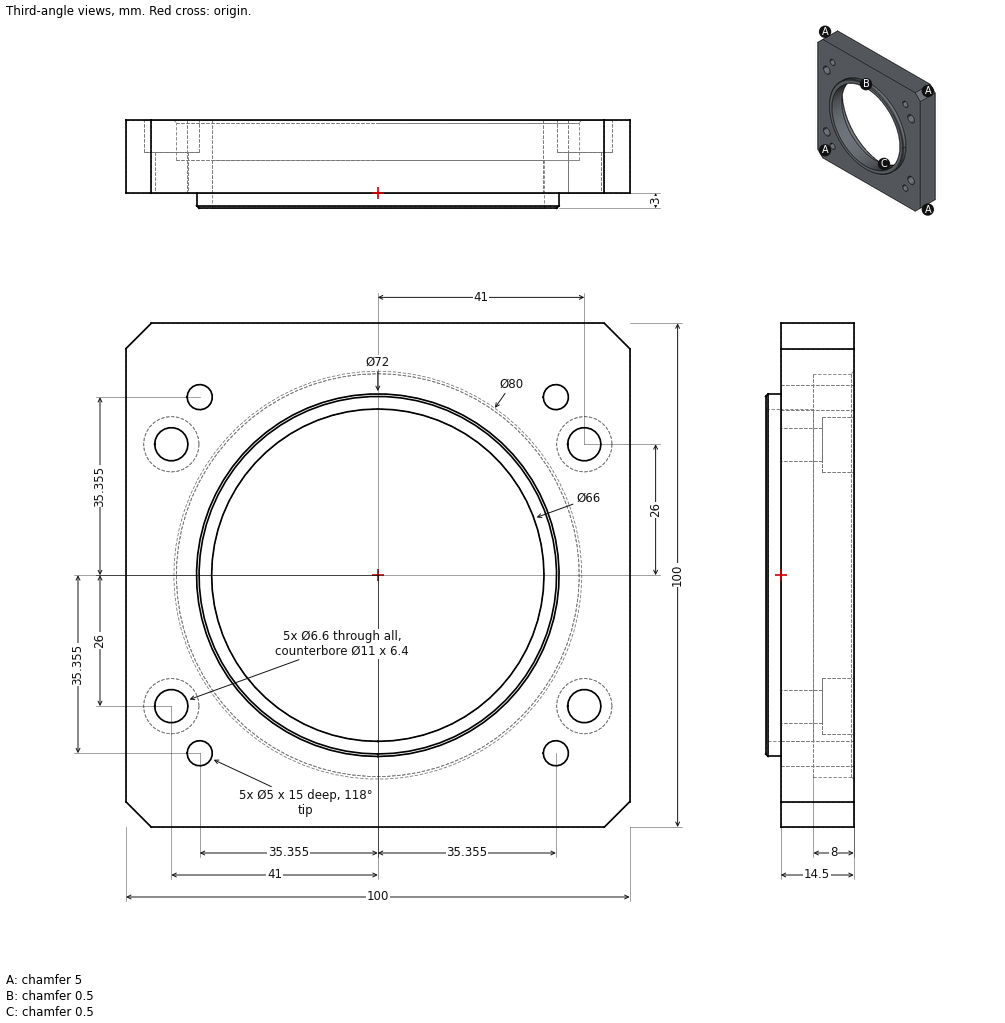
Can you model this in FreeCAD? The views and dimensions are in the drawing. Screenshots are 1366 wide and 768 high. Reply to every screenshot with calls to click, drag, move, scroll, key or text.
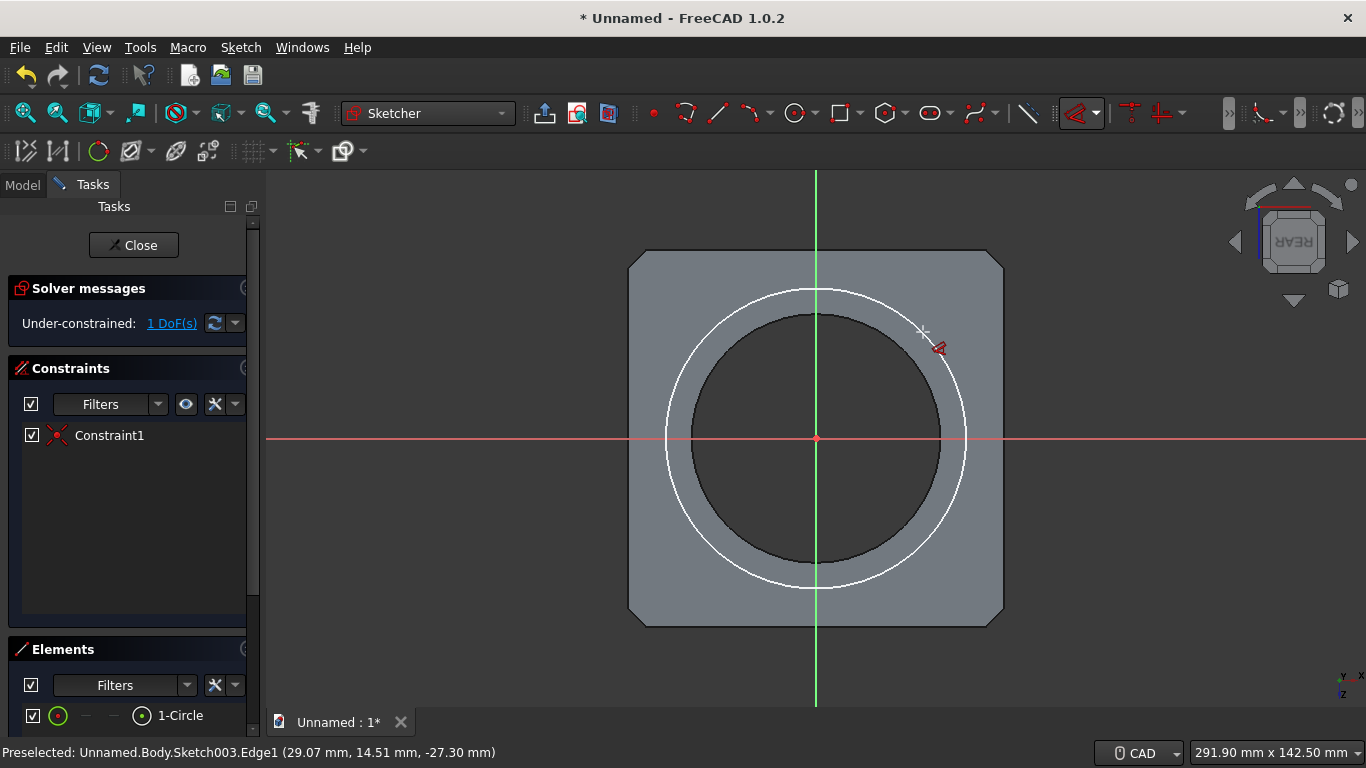
click(922, 332)
click(945, 309)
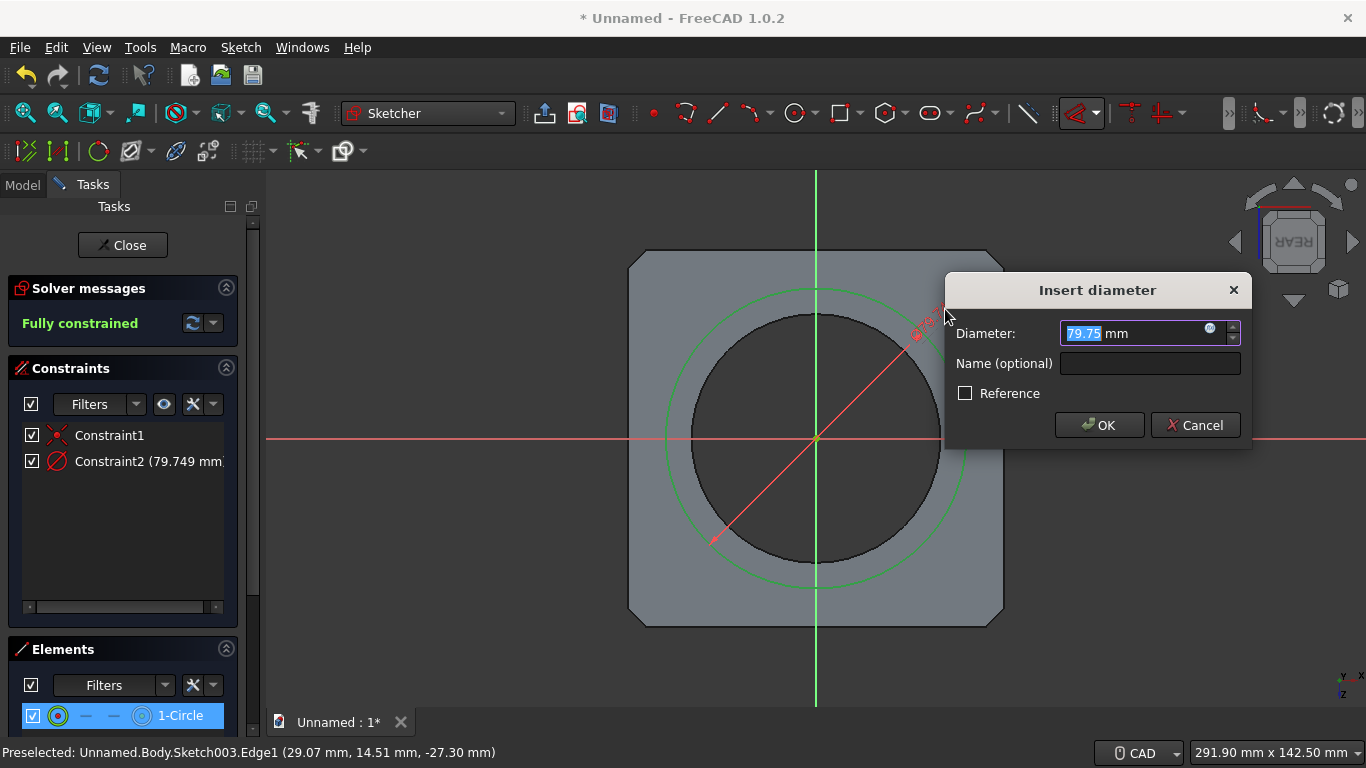
text(80)
key(Return)
key(Escape)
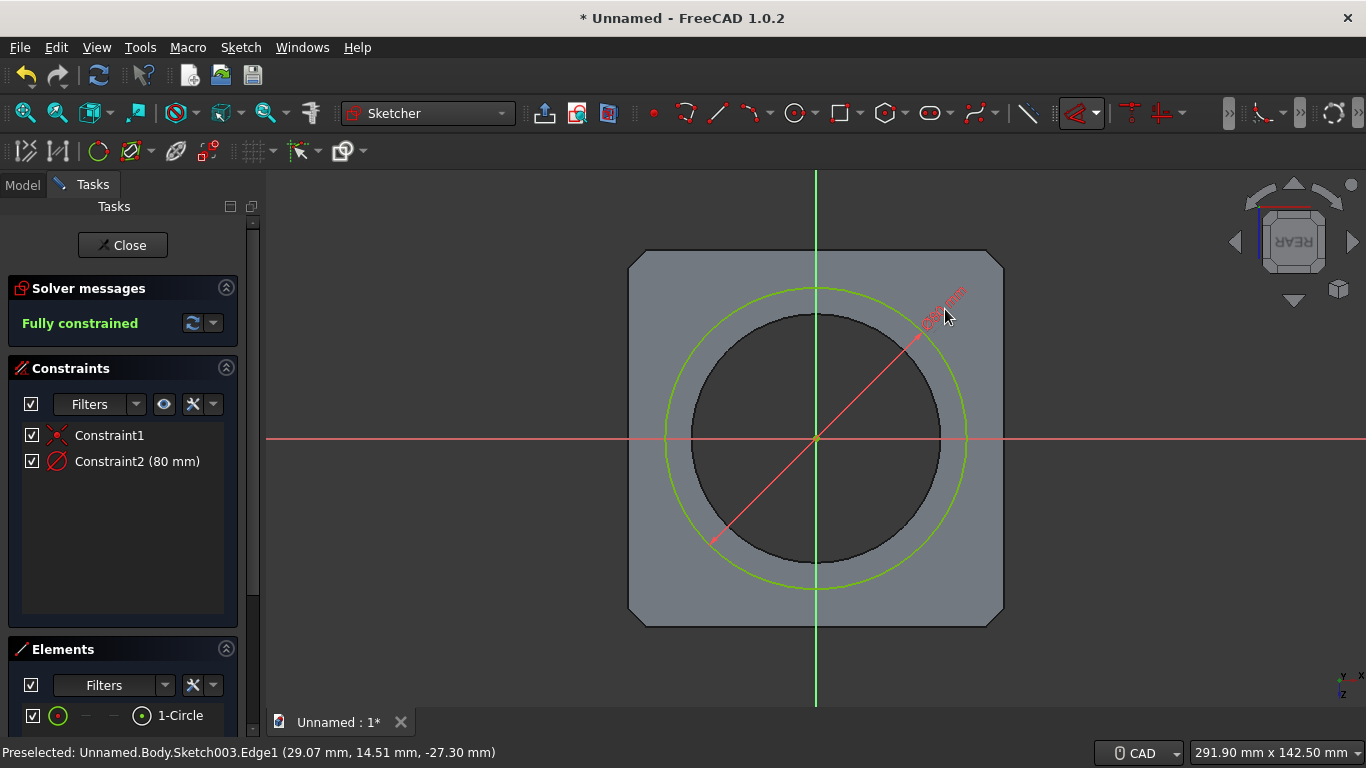
click(123, 245)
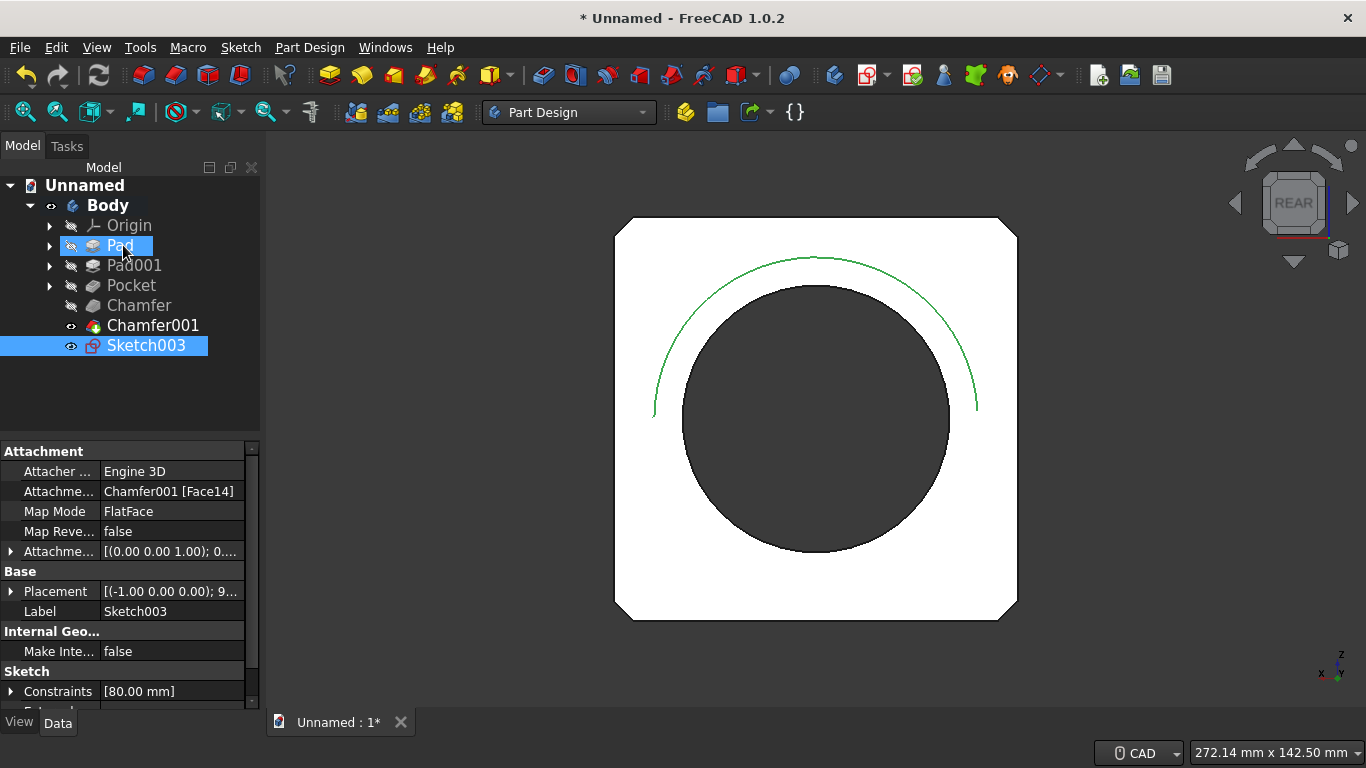
click(544, 76)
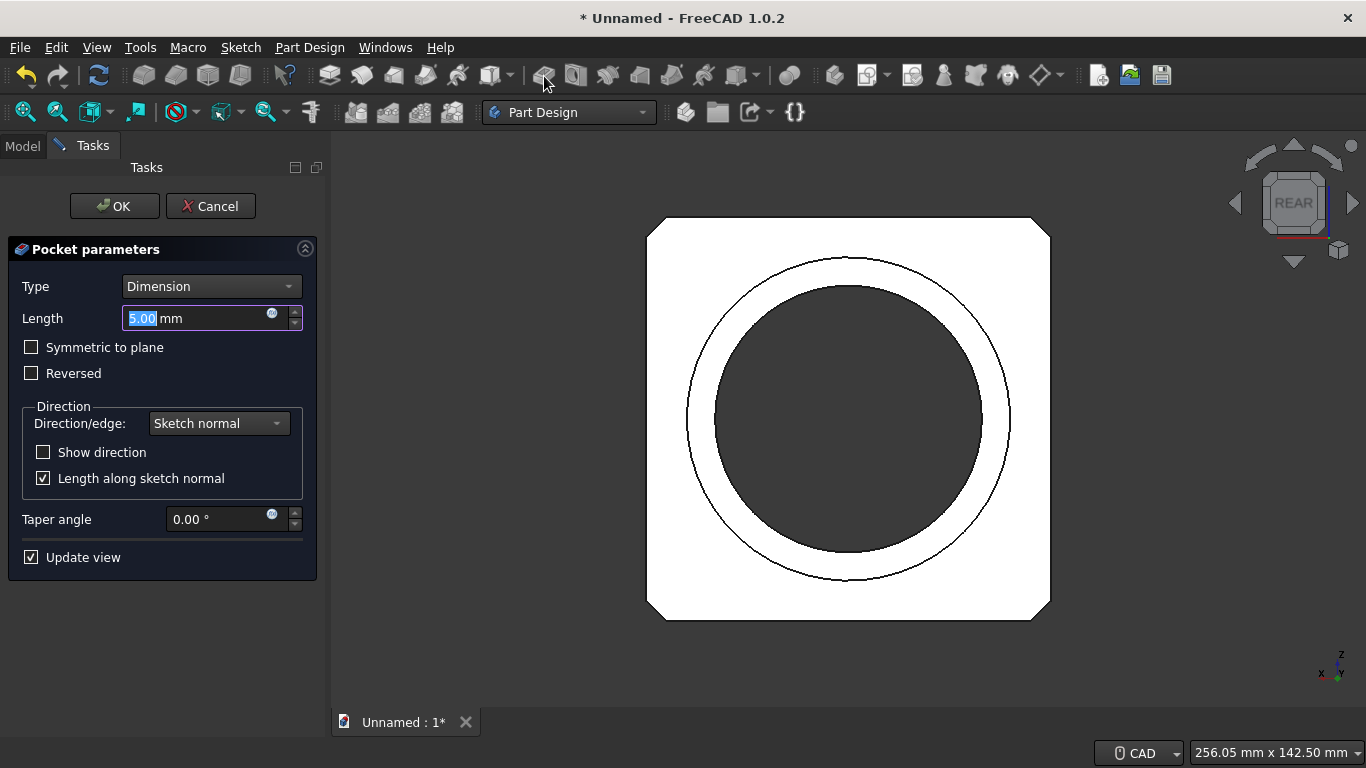
text(8)
key(Tab)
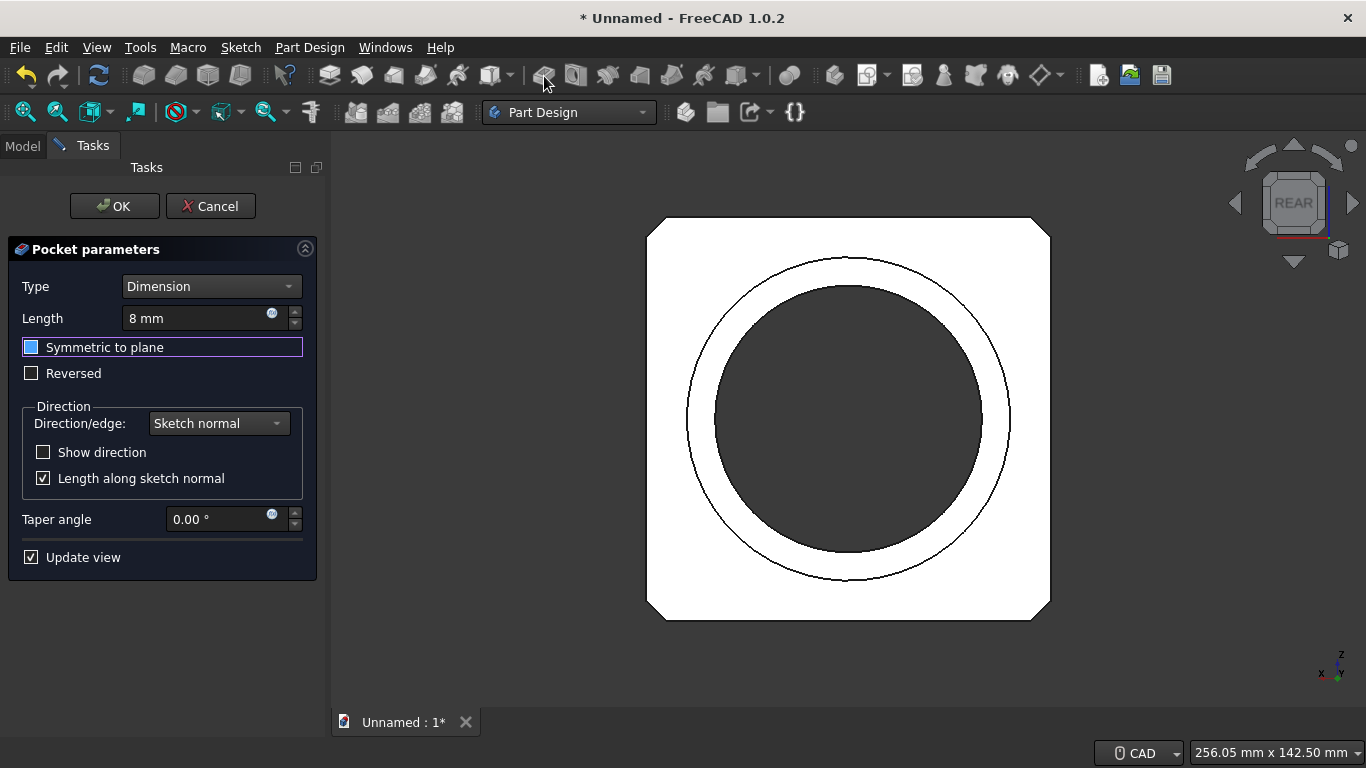
click(115, 206)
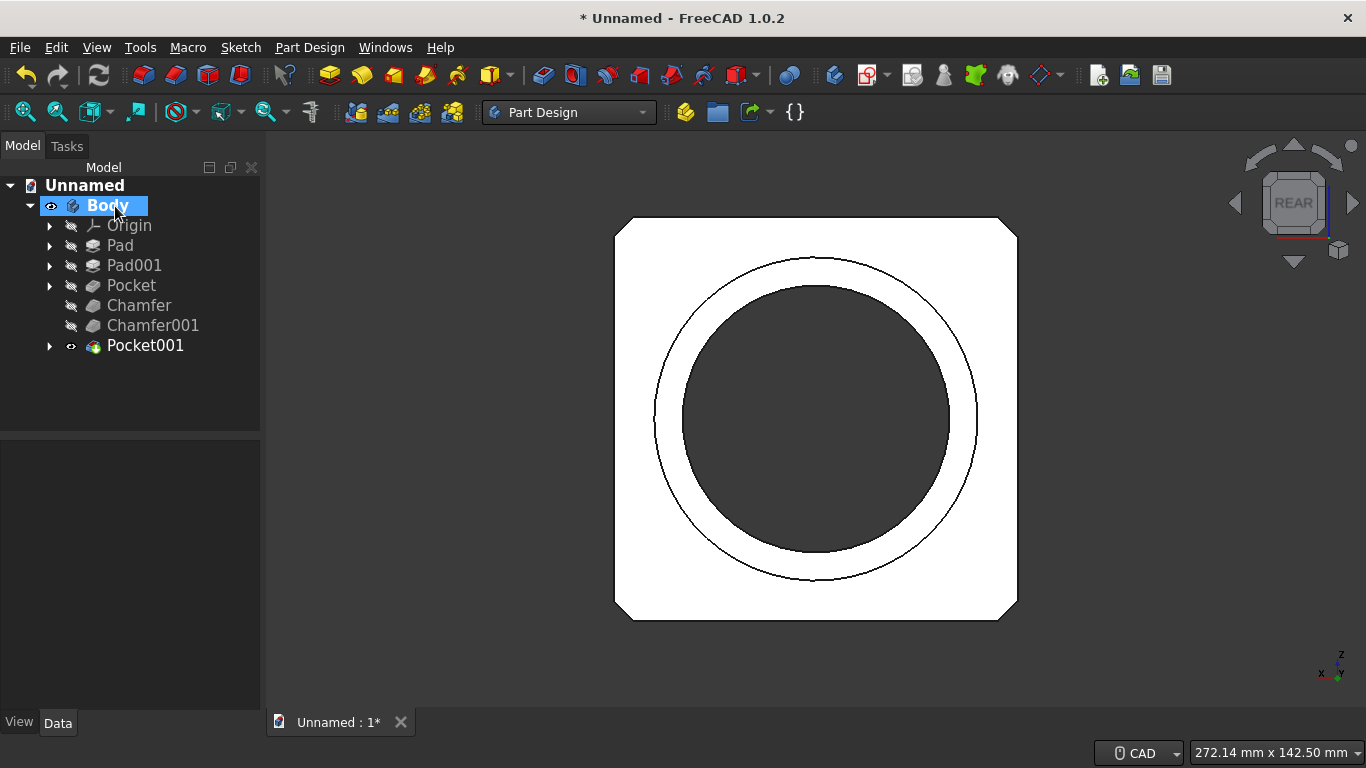
click(701, 245)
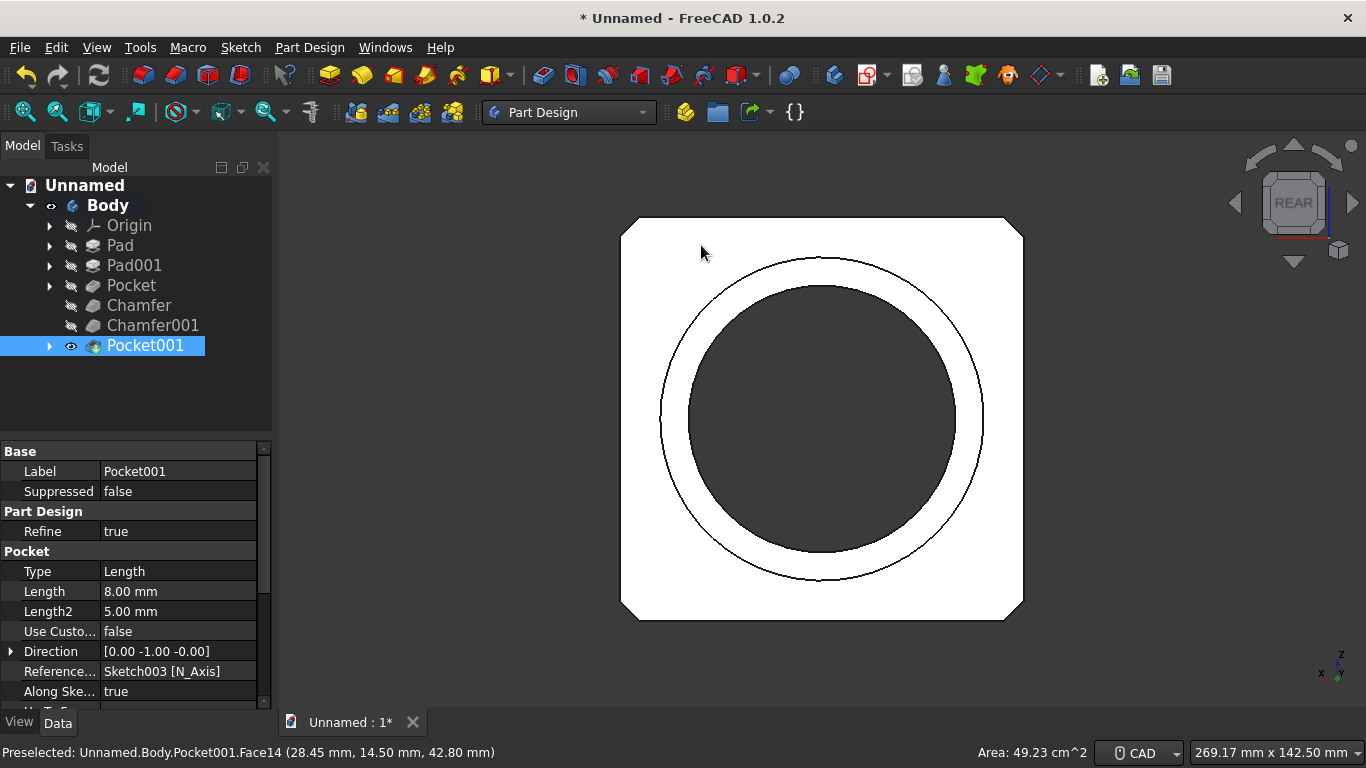
click(868, 76)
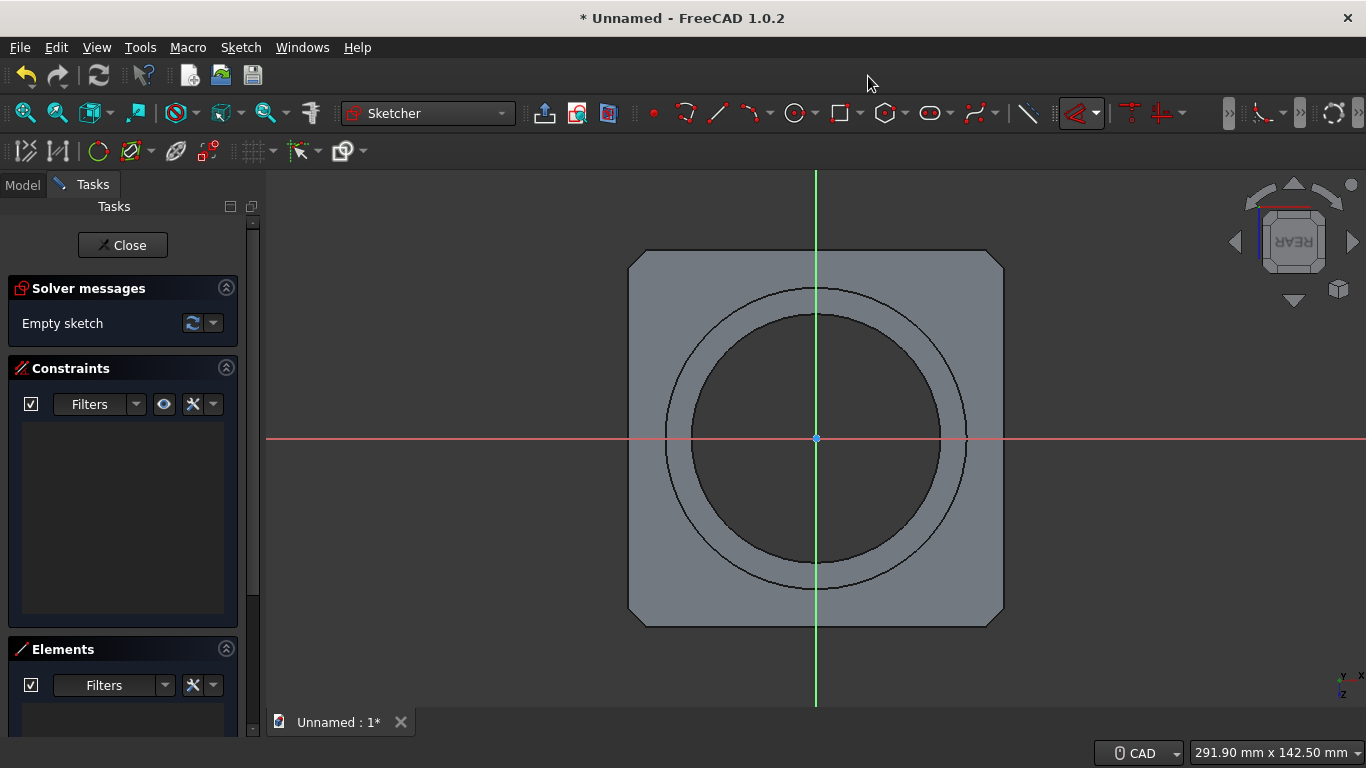
key(g)
key(c)